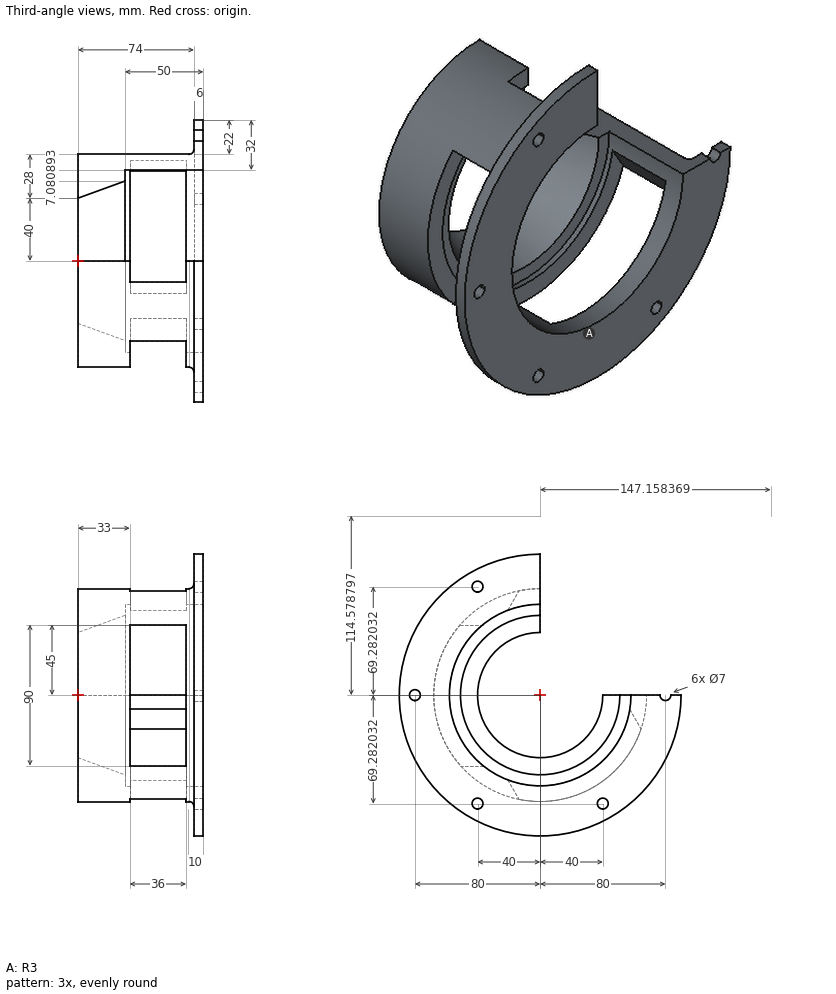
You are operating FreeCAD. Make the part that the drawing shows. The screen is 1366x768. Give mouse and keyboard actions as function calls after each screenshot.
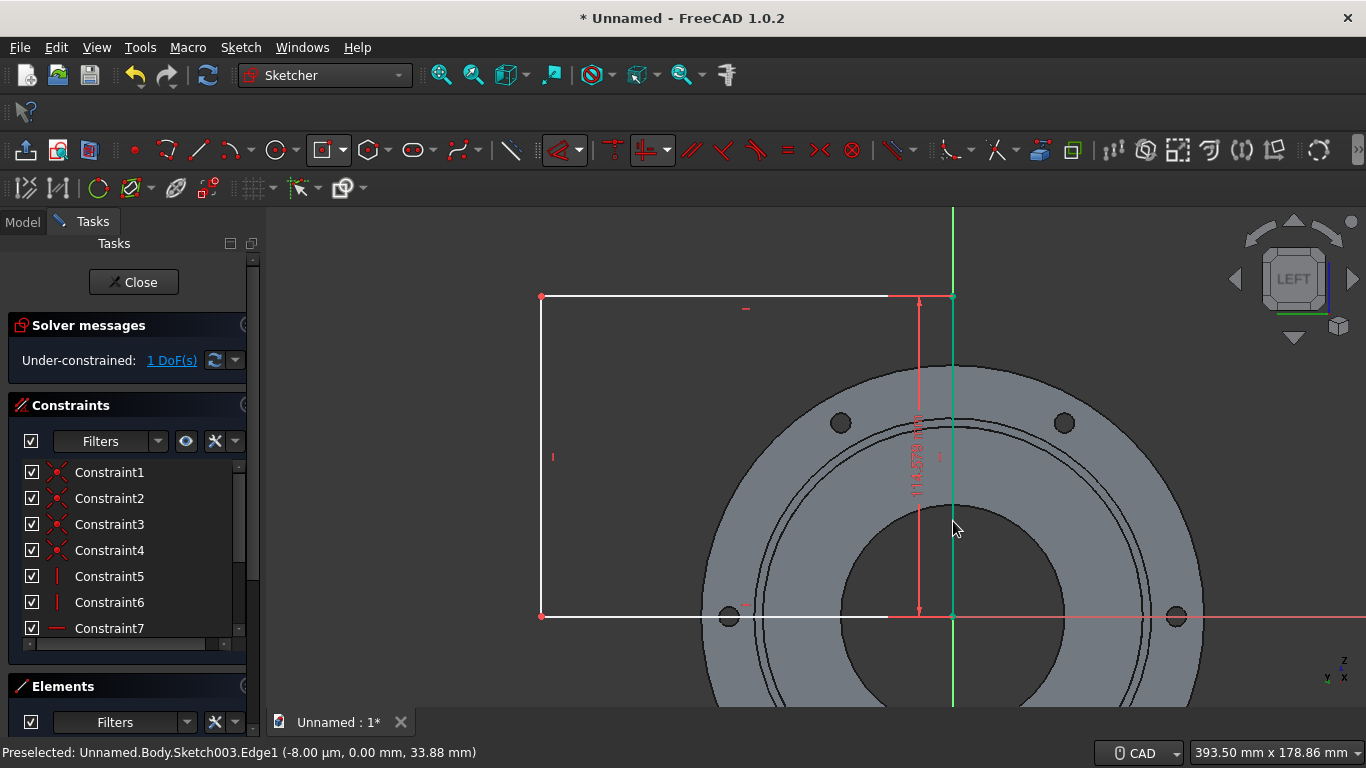
click(829, 296)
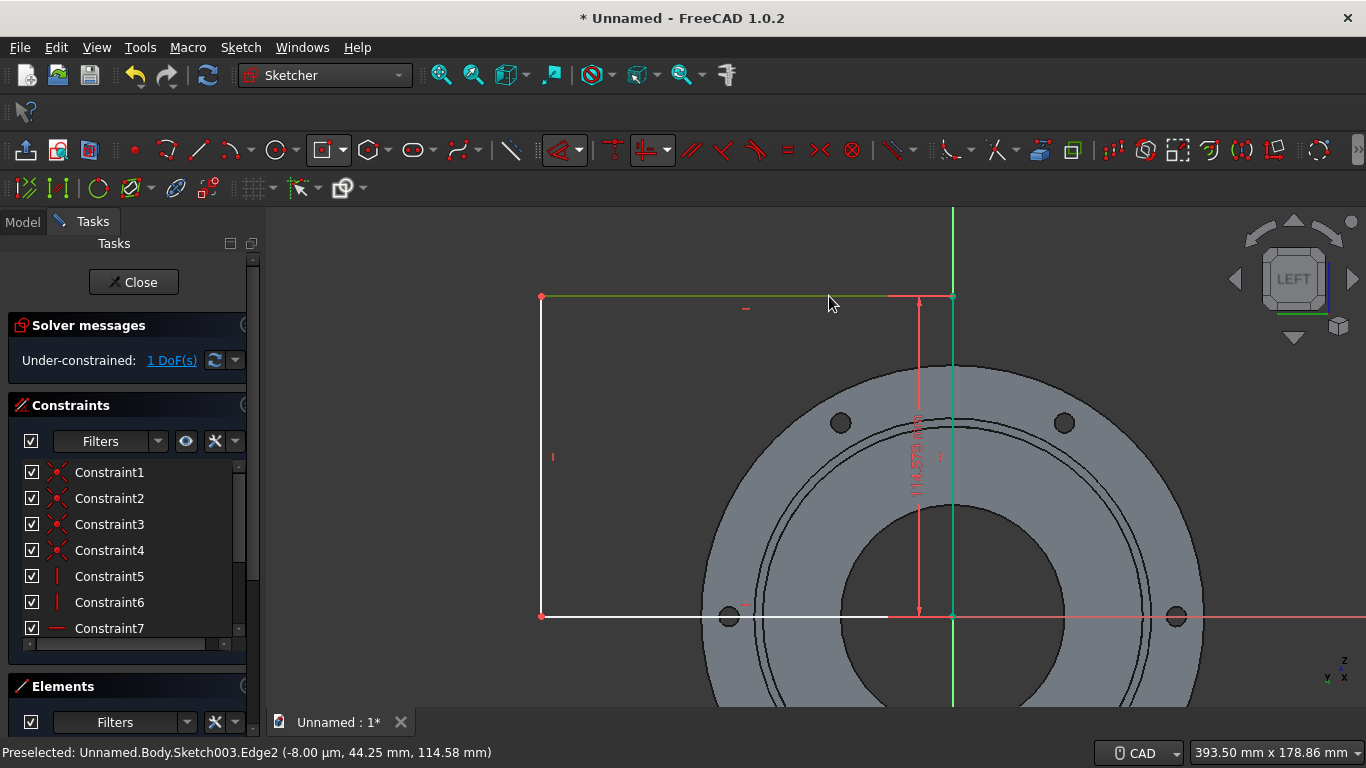
key(l)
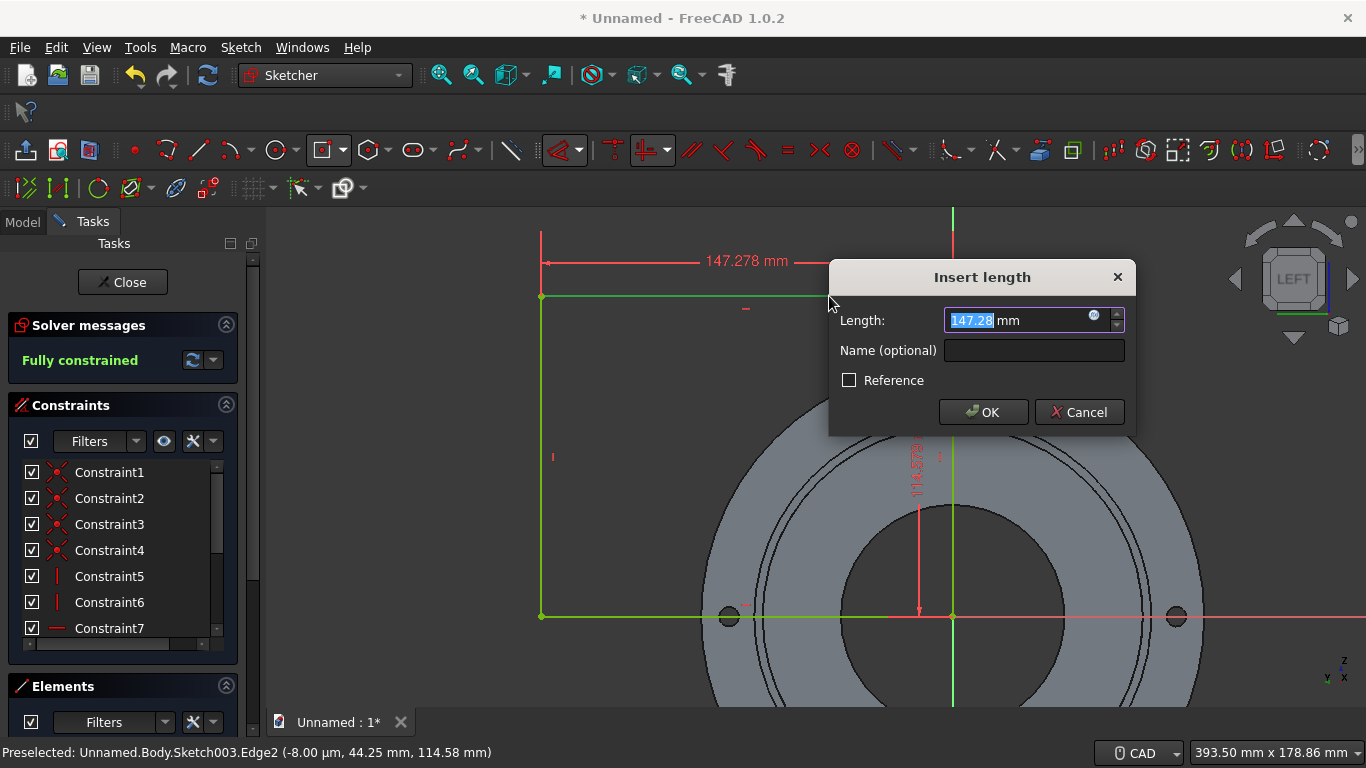
text(147.158369)
key(Return)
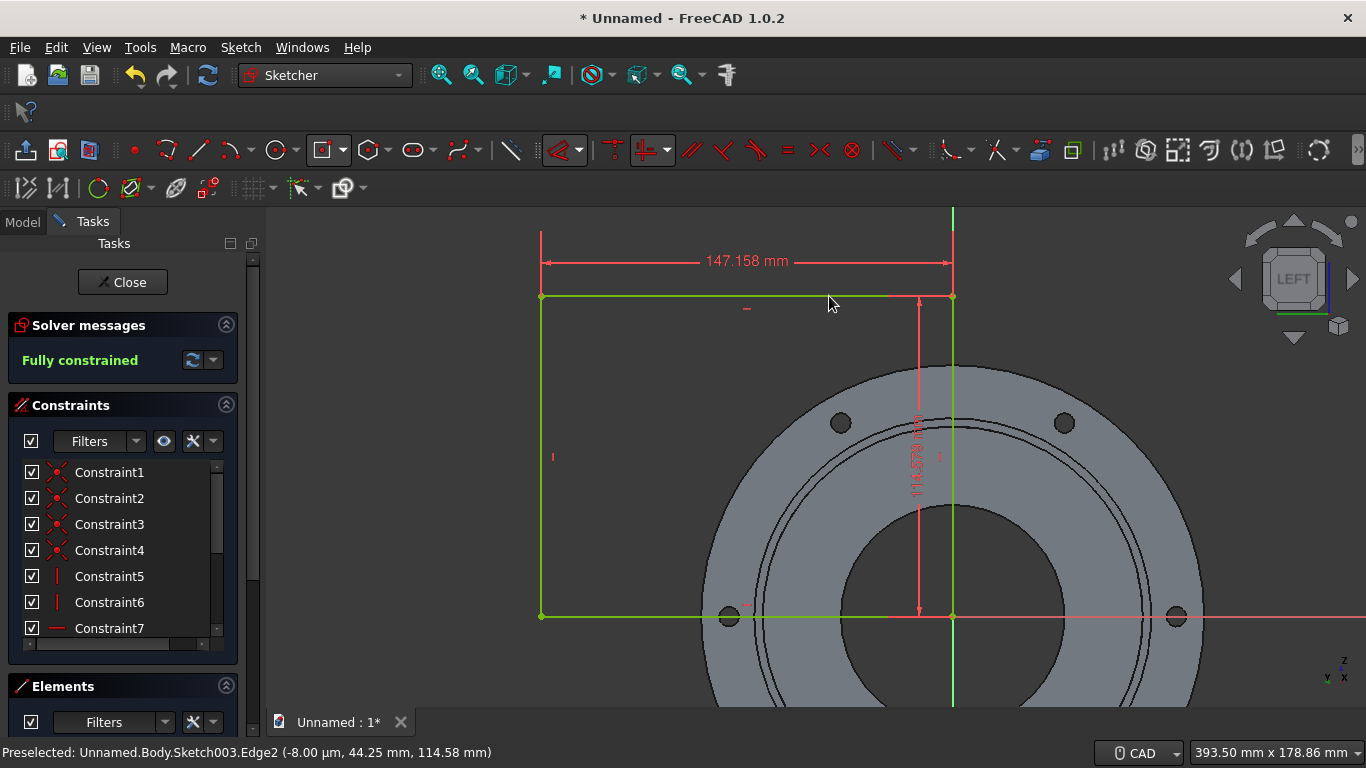
click(123, 282)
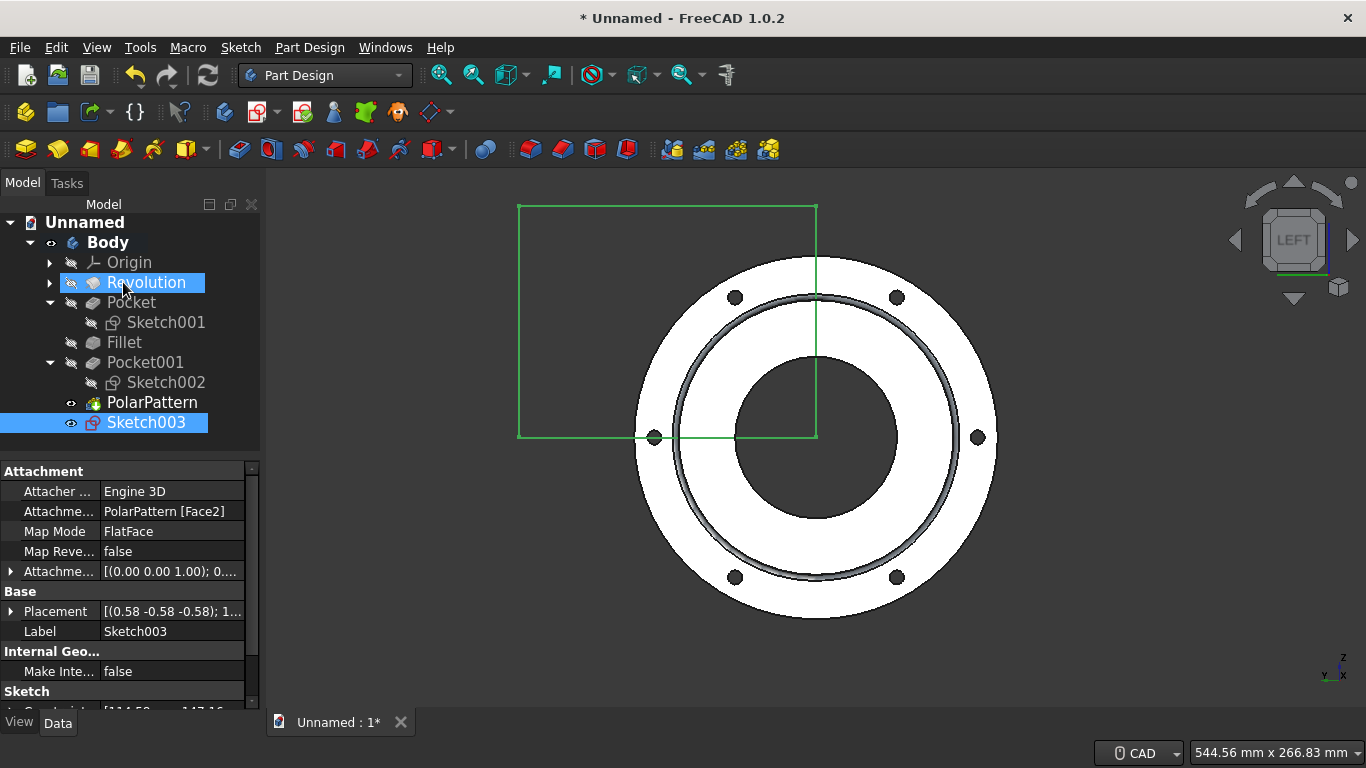
click(240, 150)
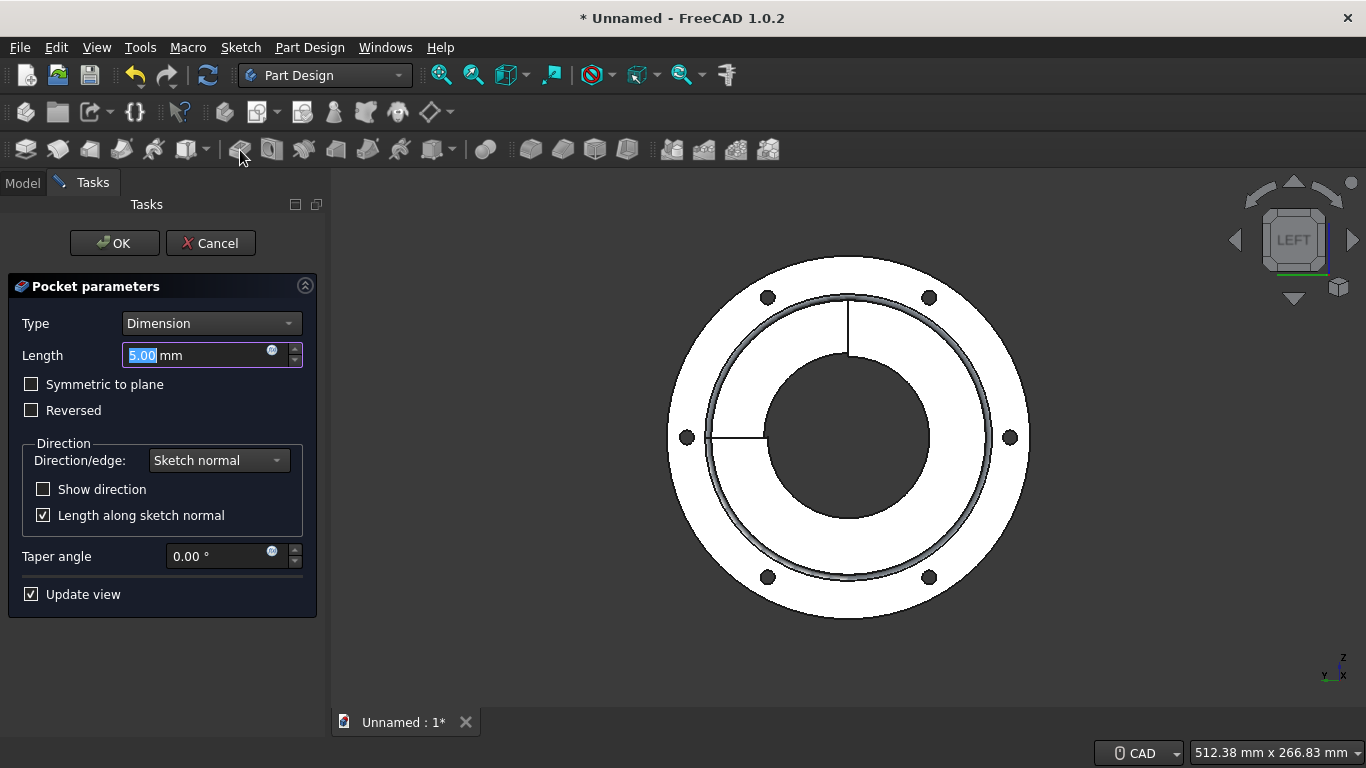
click(212, 324)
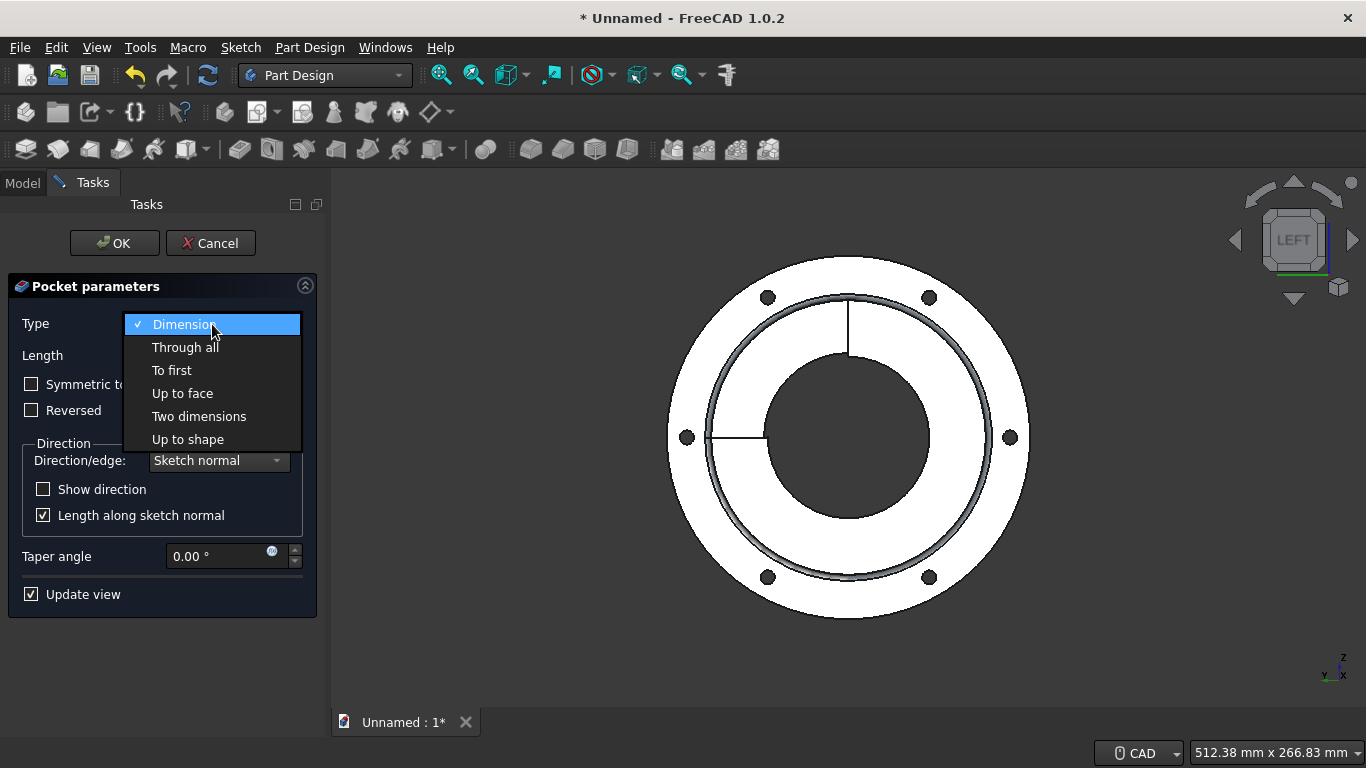
click(212, 348)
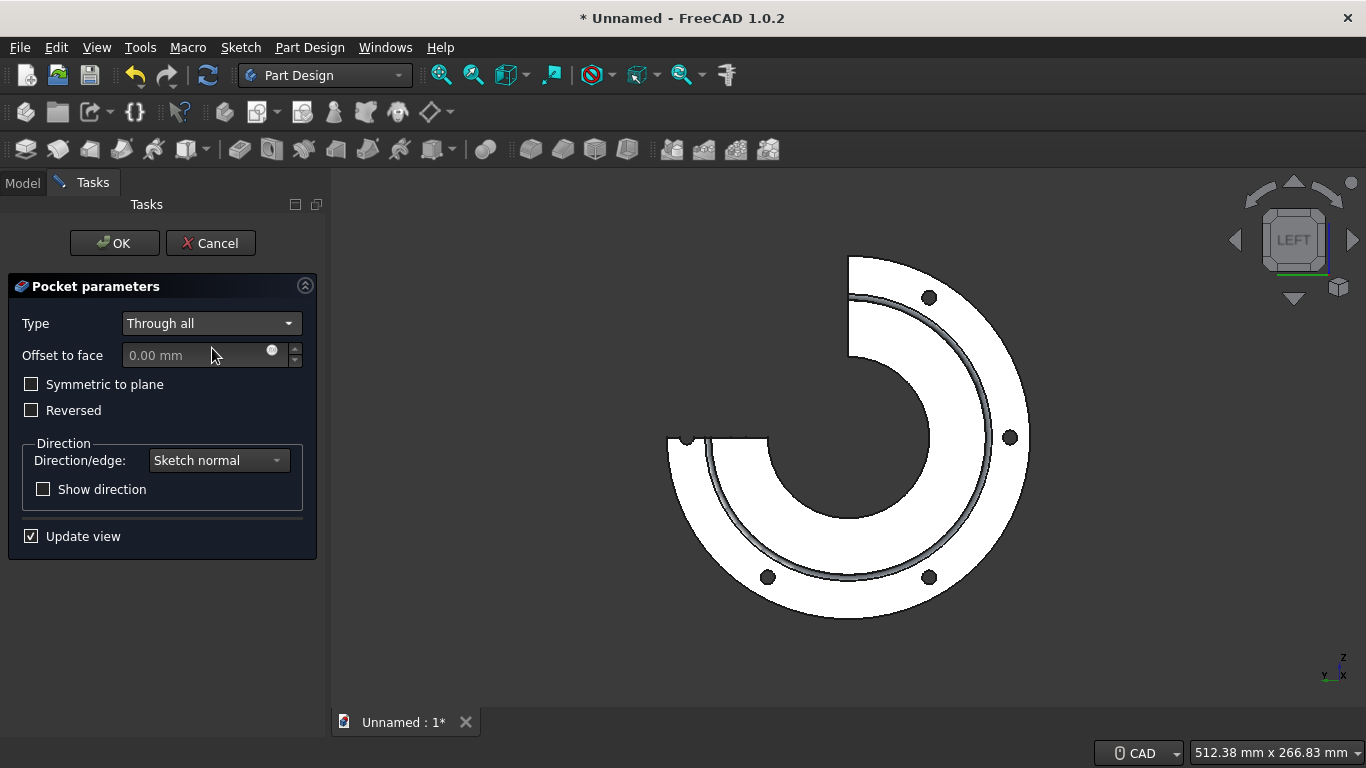
click(115, 243)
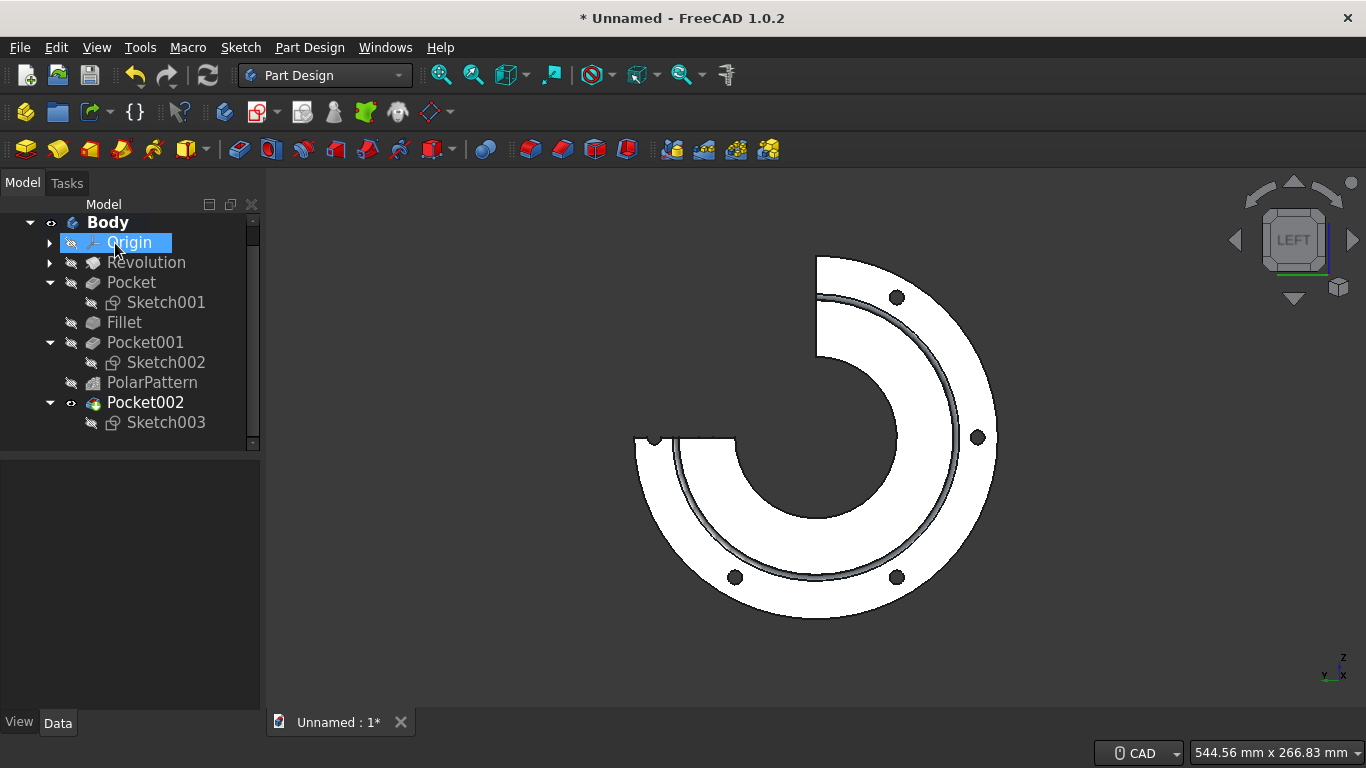
key(0)